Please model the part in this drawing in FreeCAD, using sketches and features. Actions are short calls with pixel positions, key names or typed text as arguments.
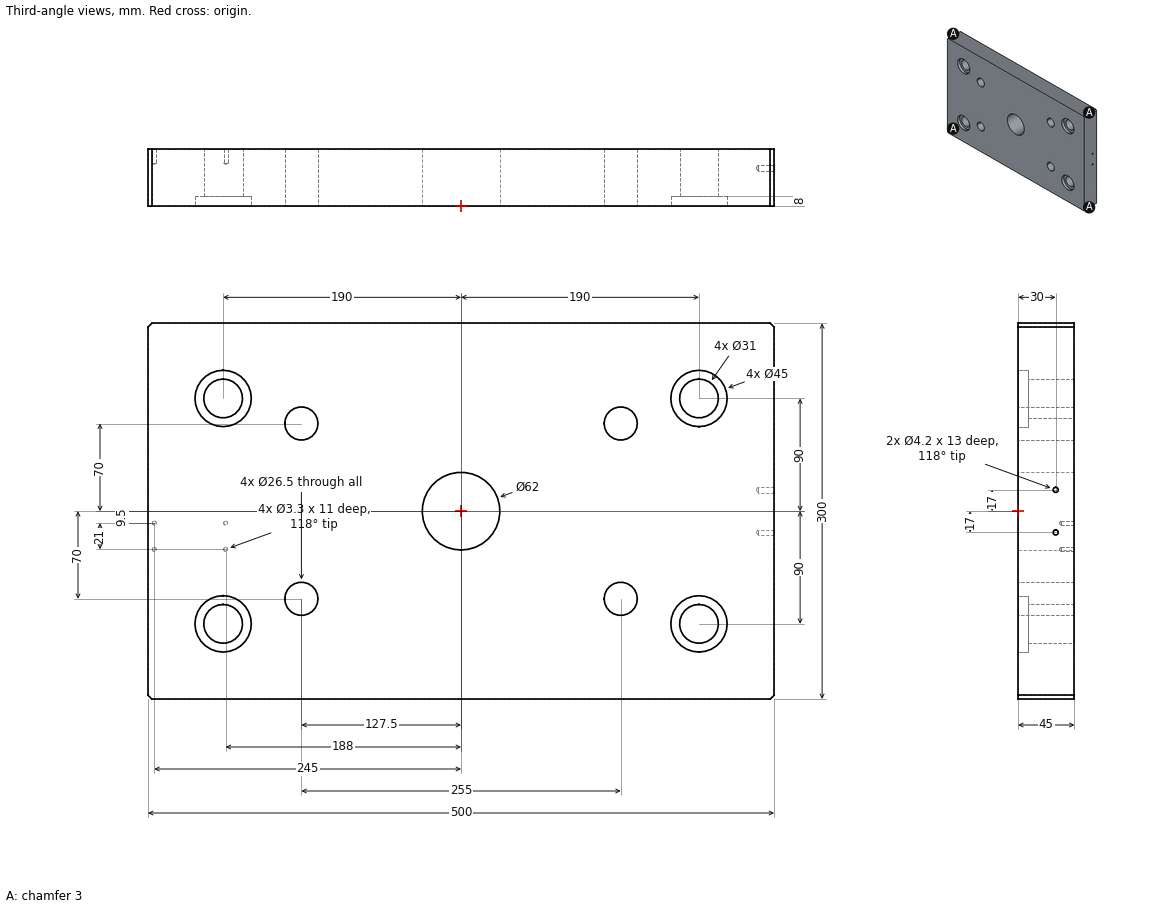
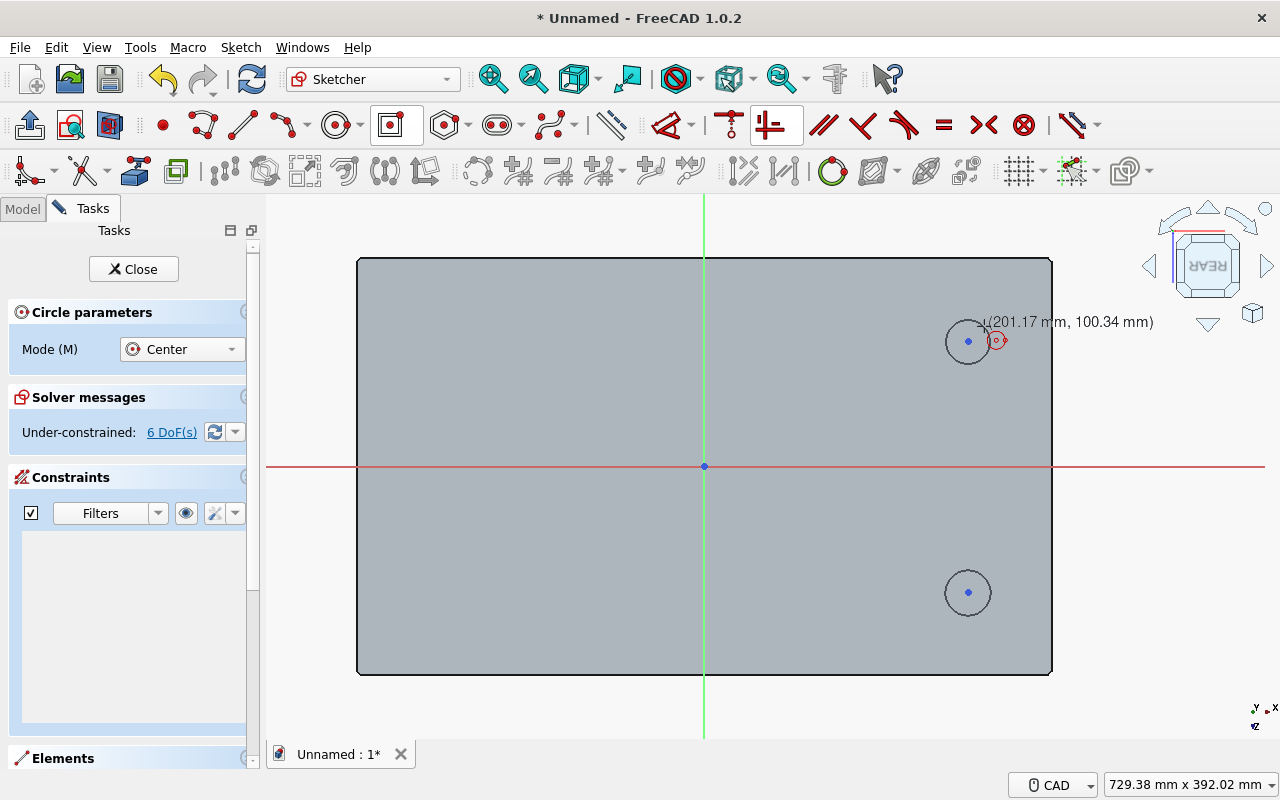
click(440, 341)
click(455, 326)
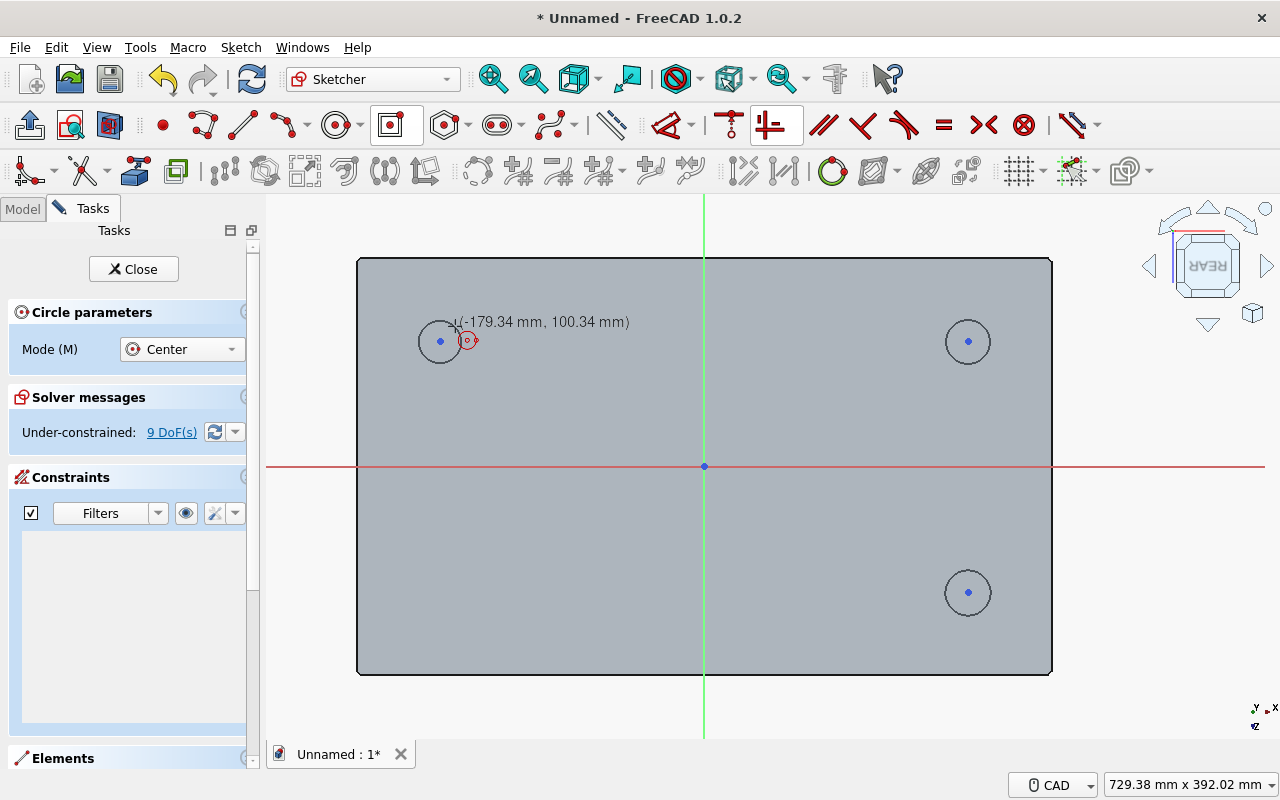
click(440, 592)
click(455, 576)
key(Escape)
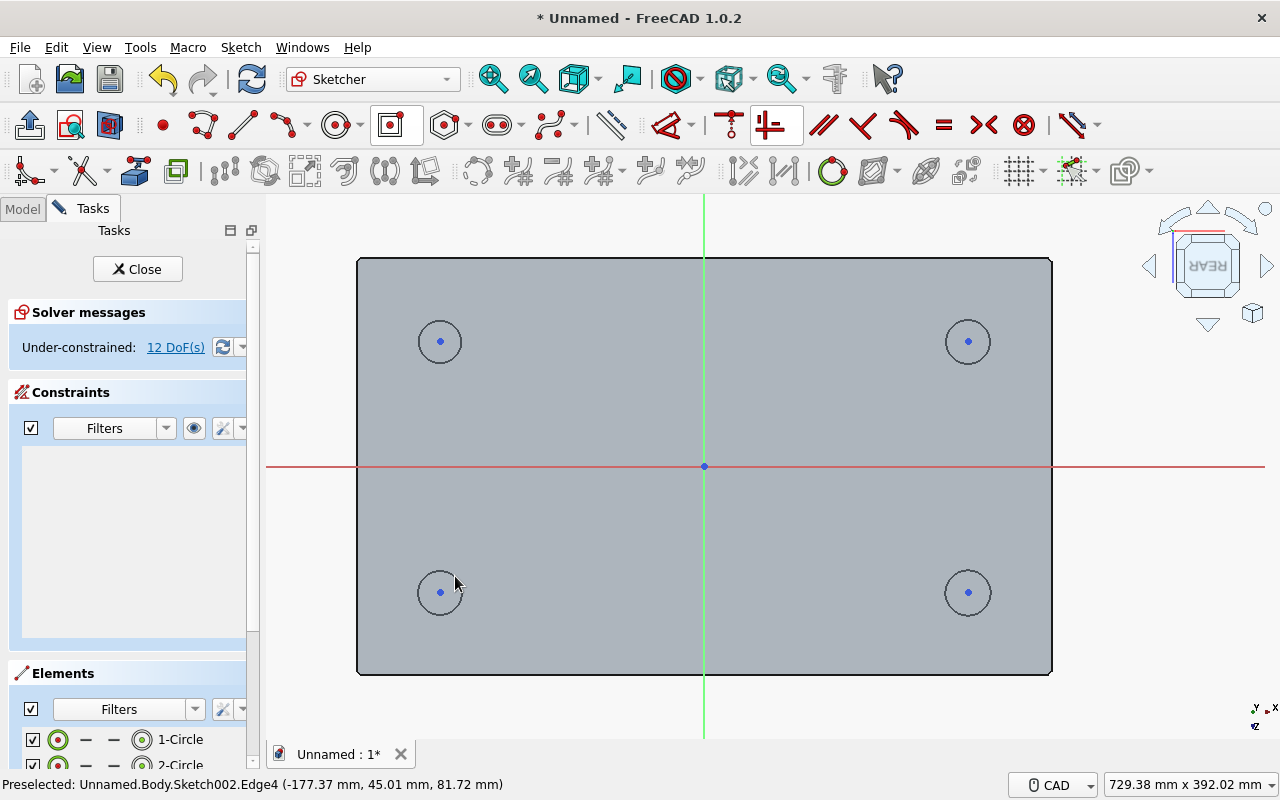
click(984, 577)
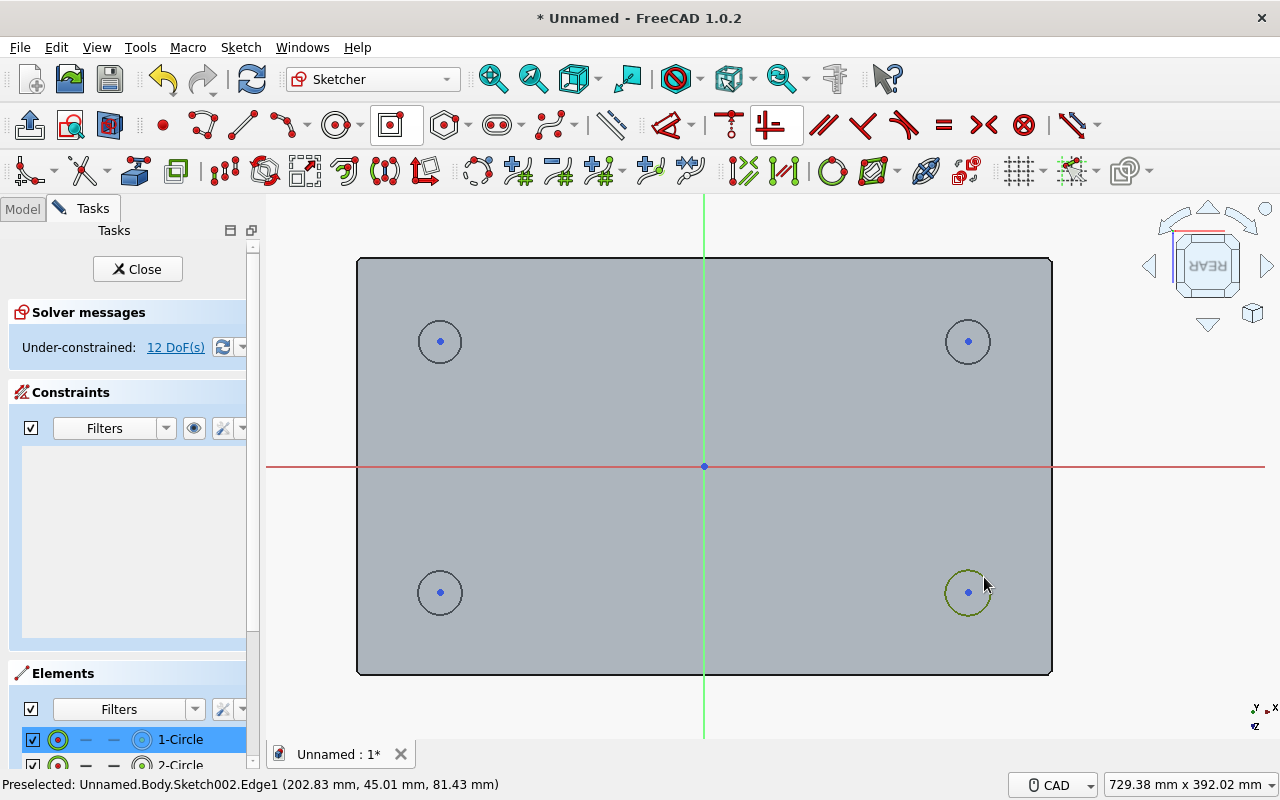
click(983, 326)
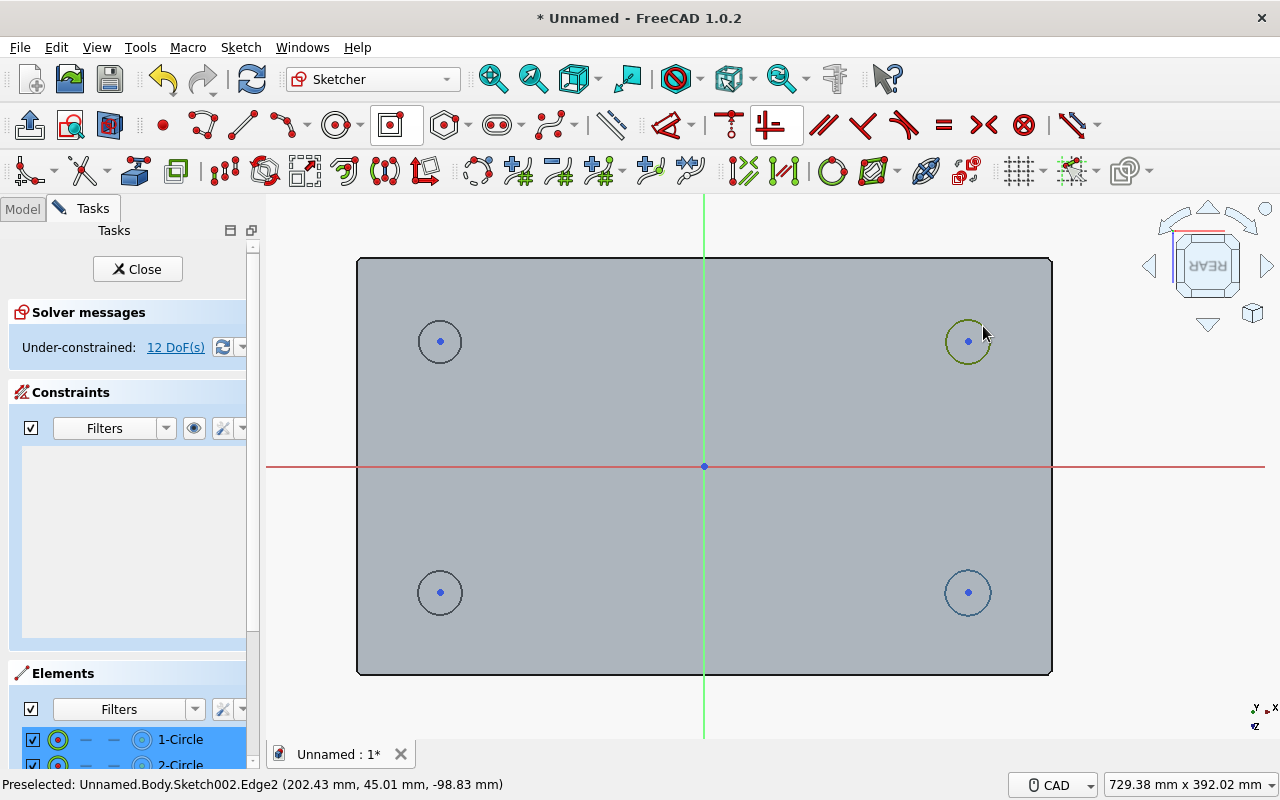
click(455, 327)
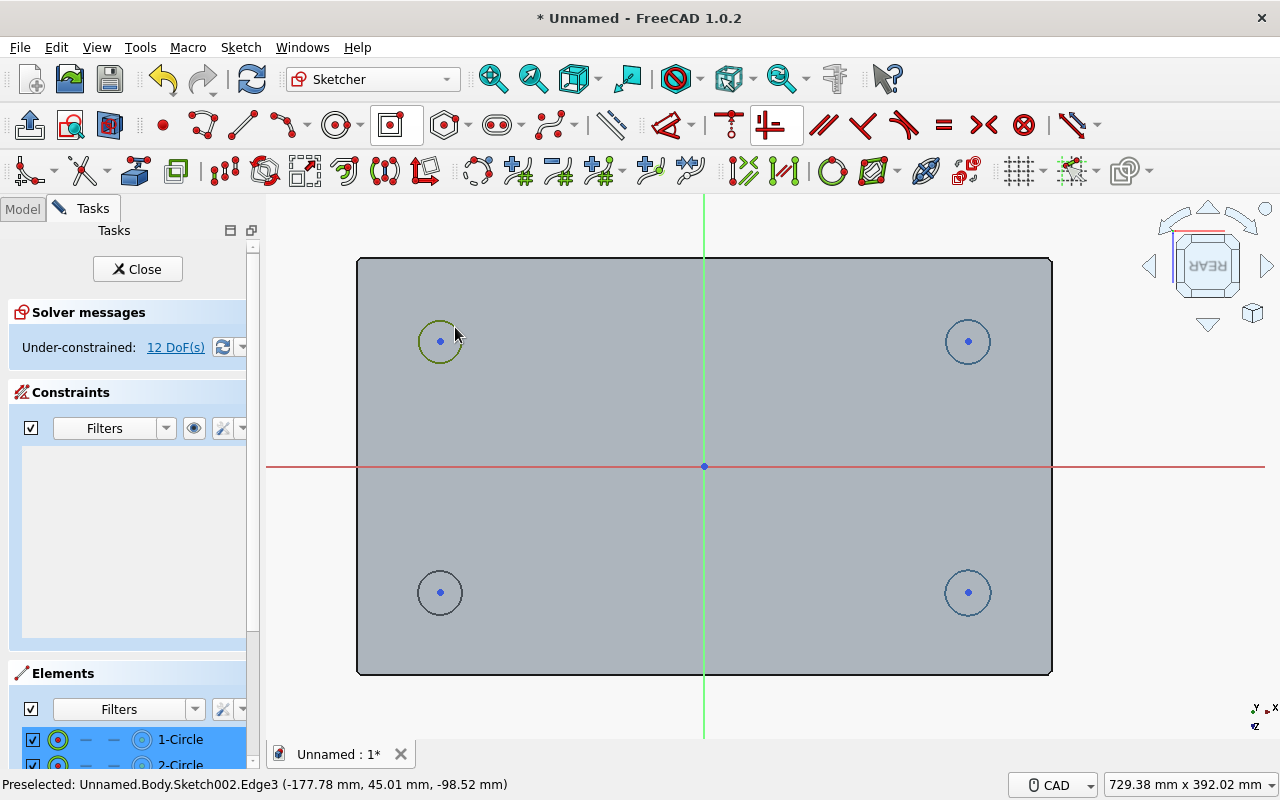
click(455, 577)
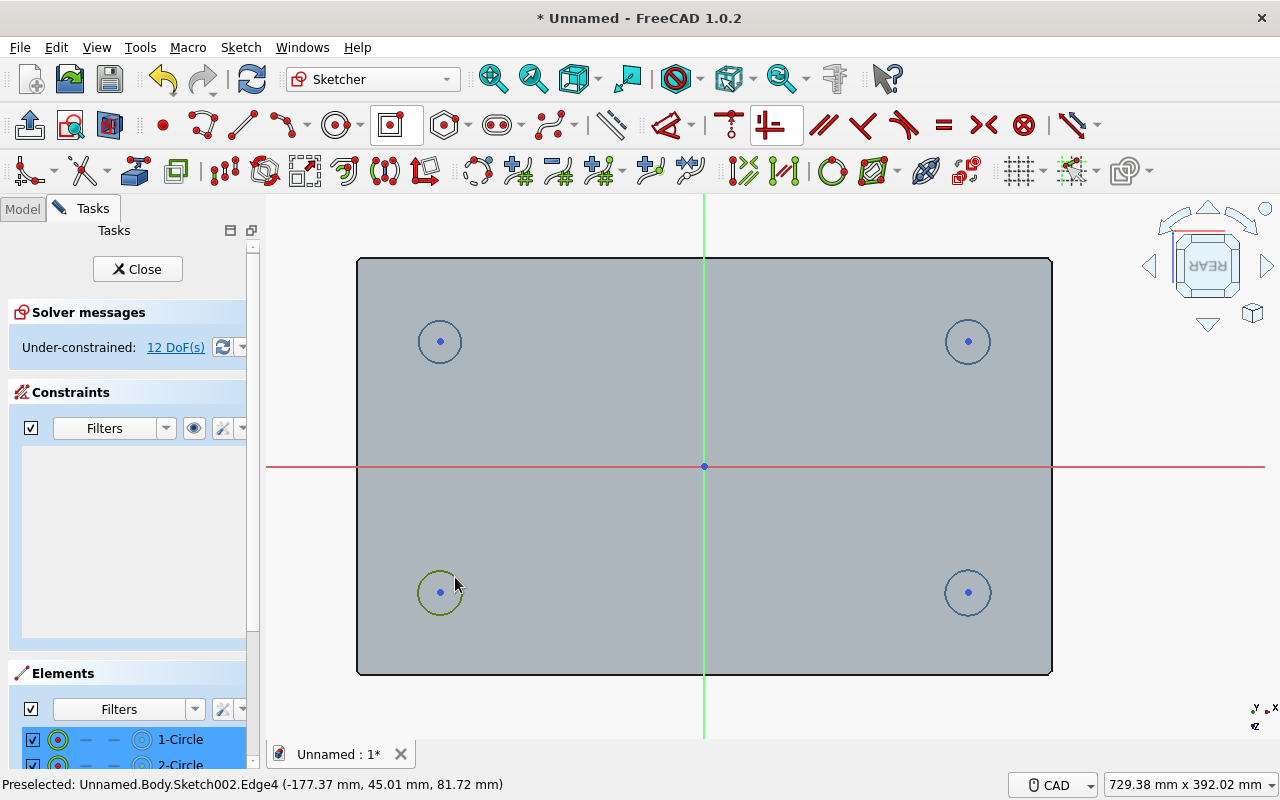
click(944, 126)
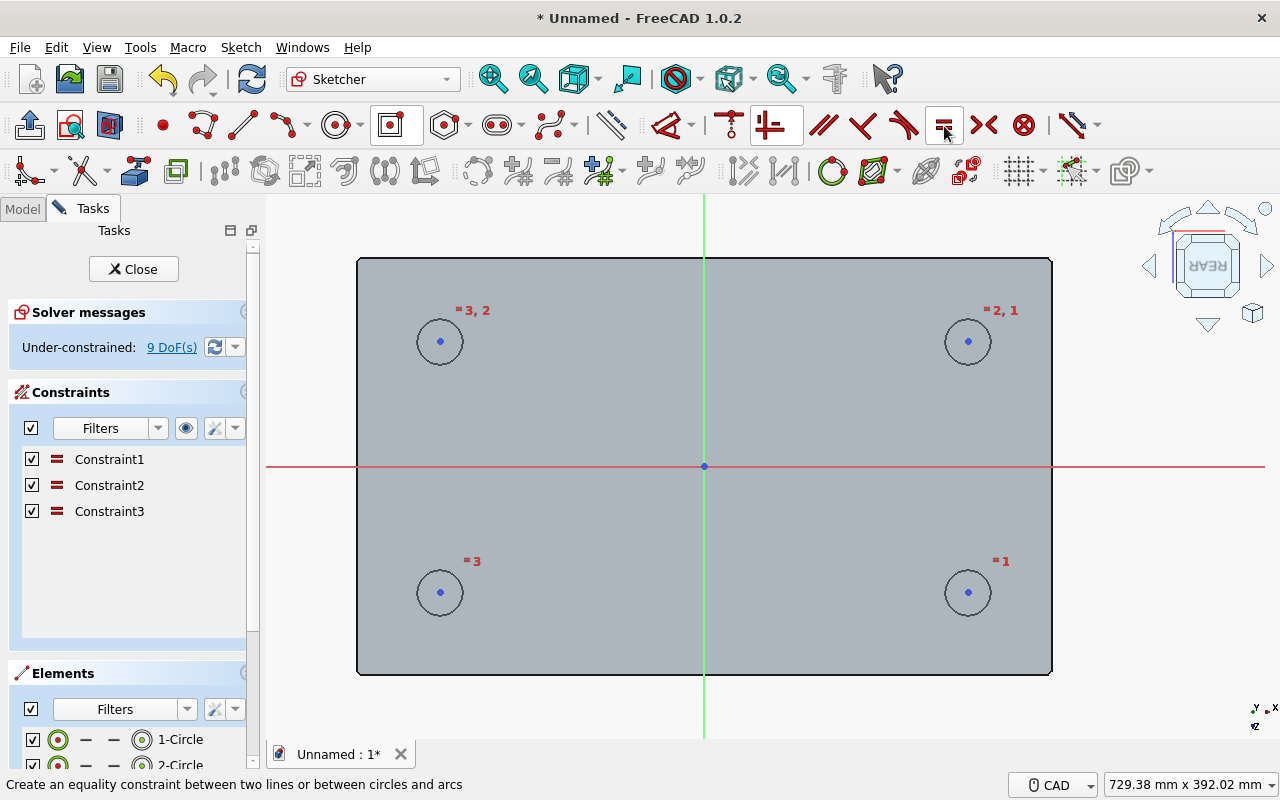
click(968, 593)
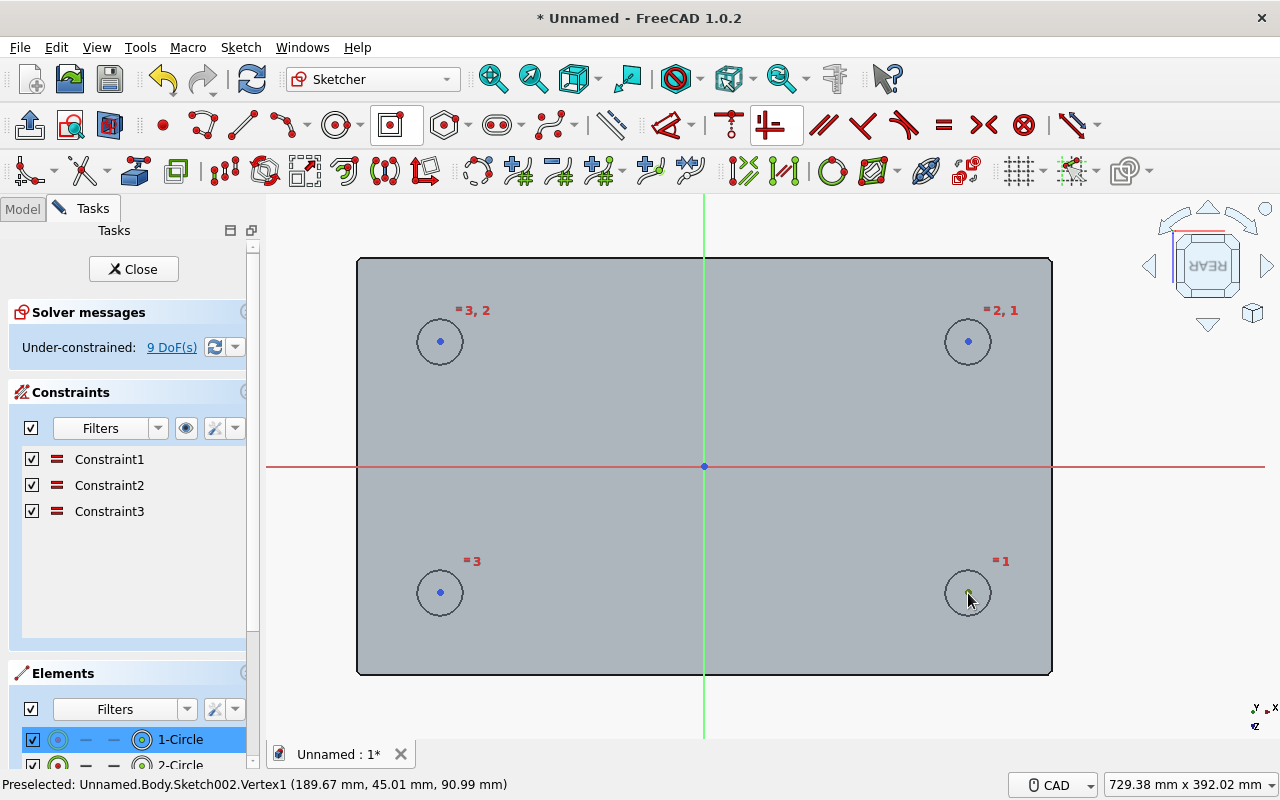
click(968, 342)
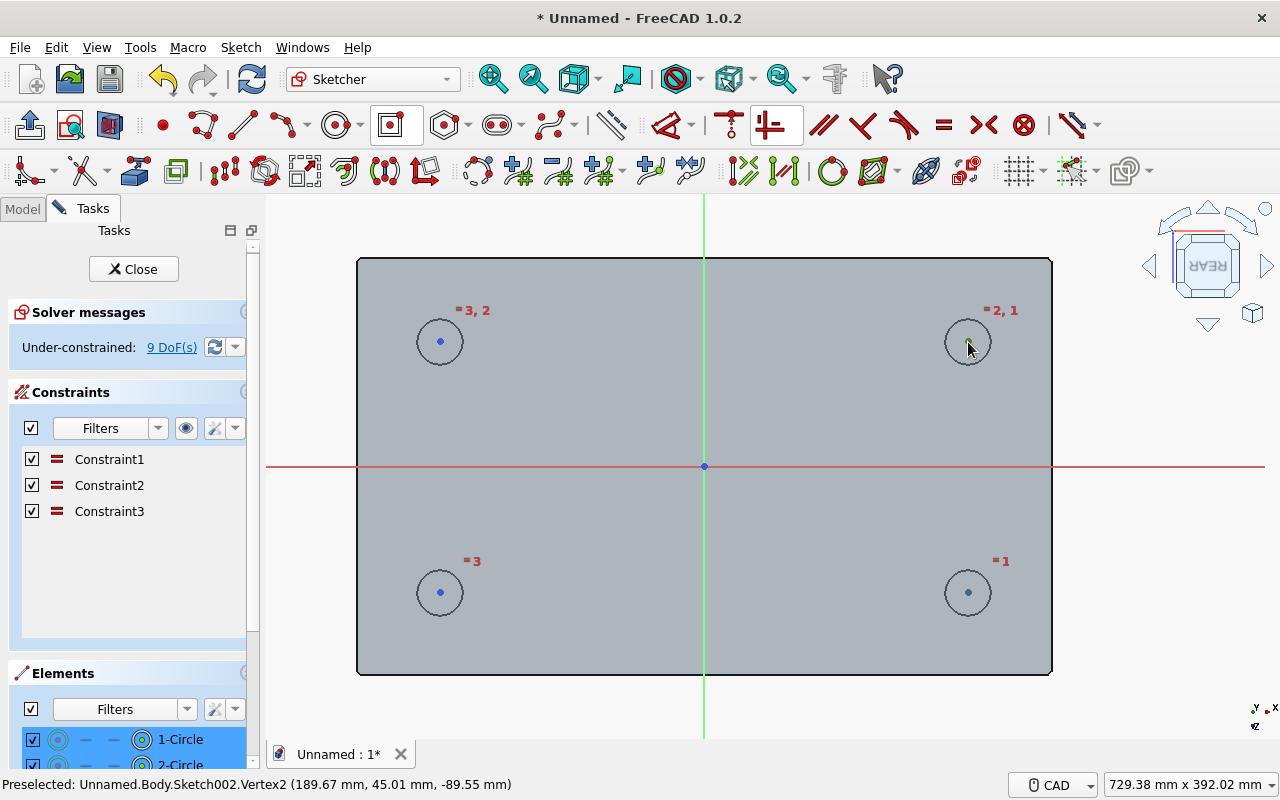
key(v)